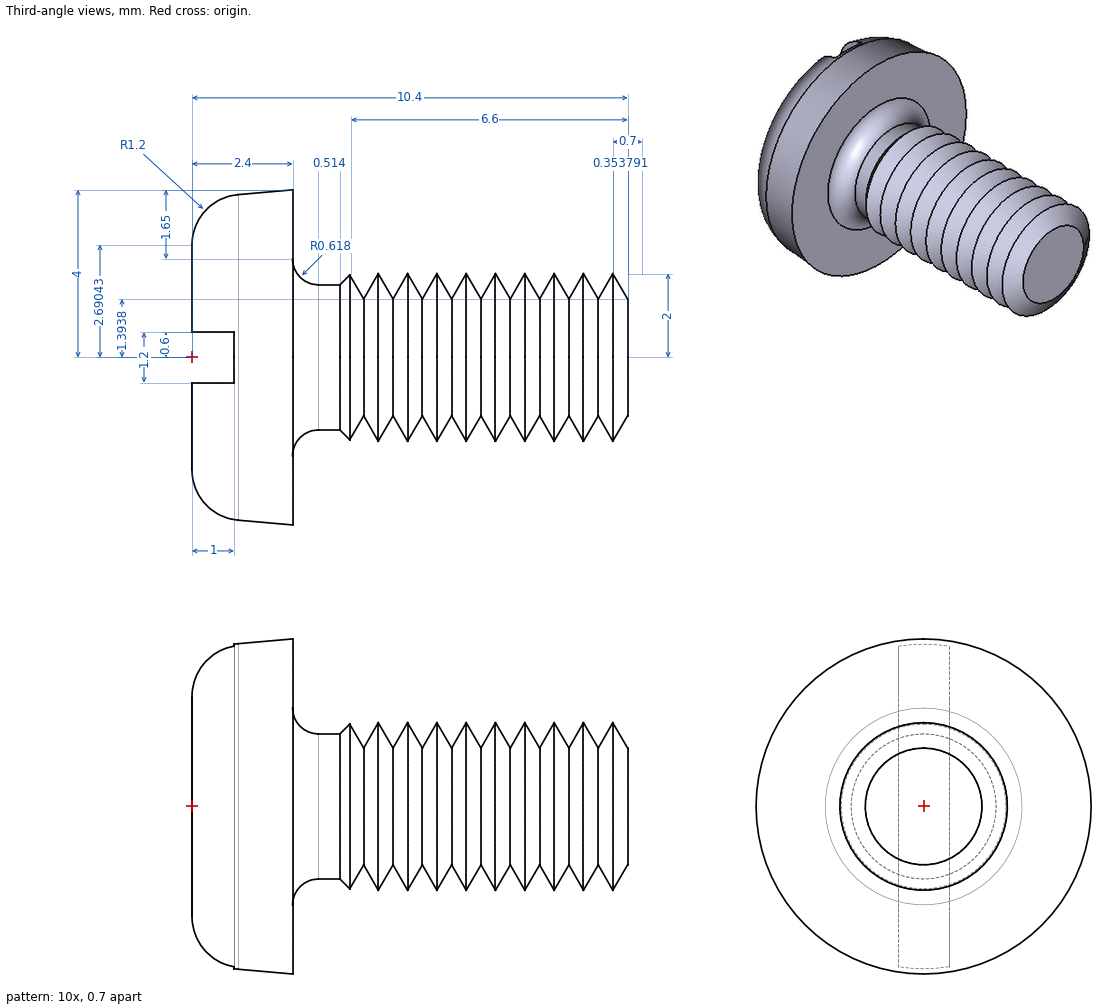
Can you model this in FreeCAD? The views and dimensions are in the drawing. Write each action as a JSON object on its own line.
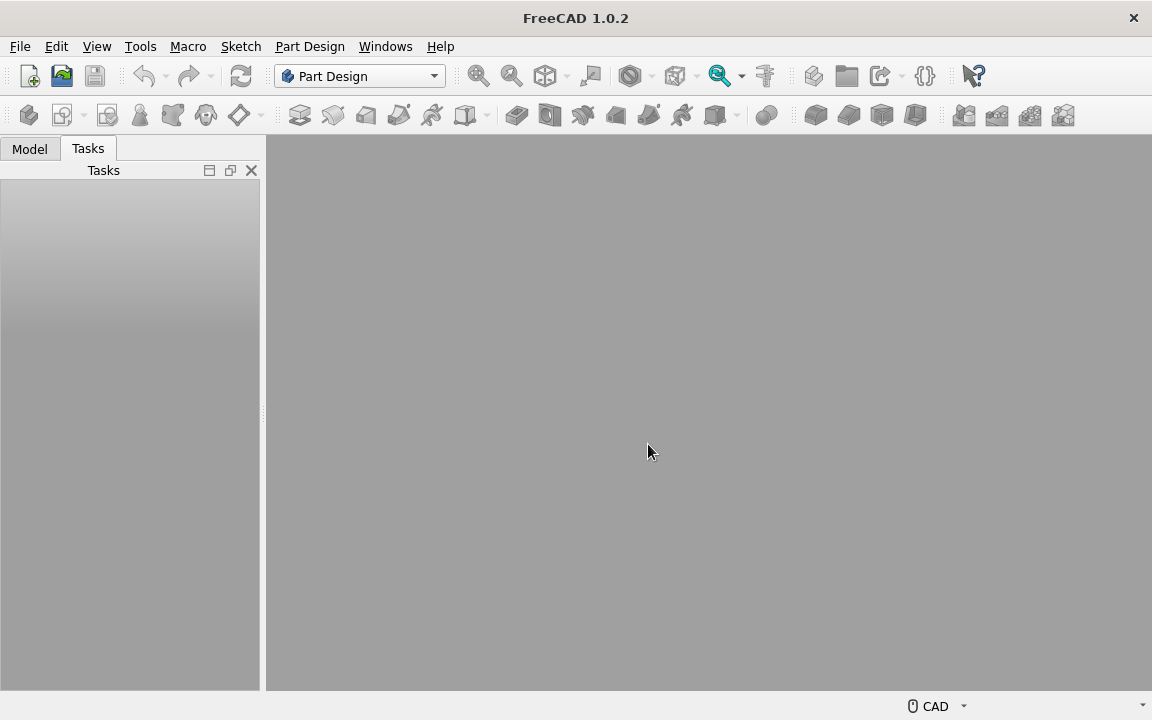
{"action": "left_click", "coordinate": [29, 76]}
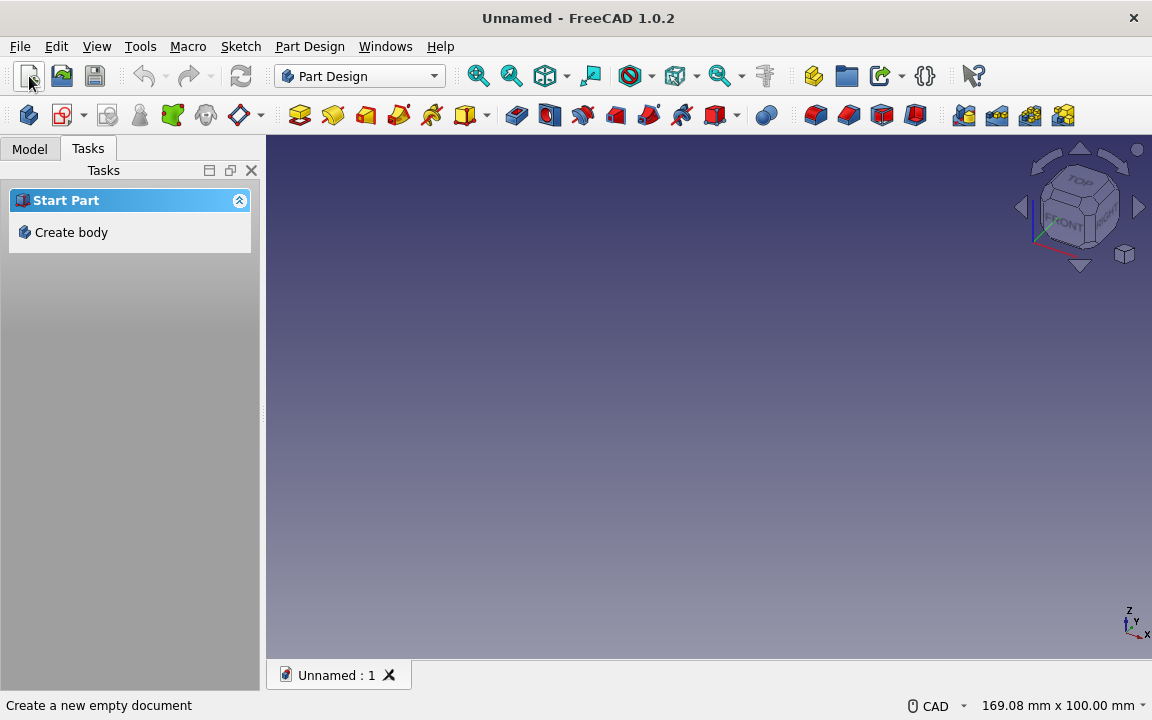
{"action": "left_click", "coordinate": [62, 116]}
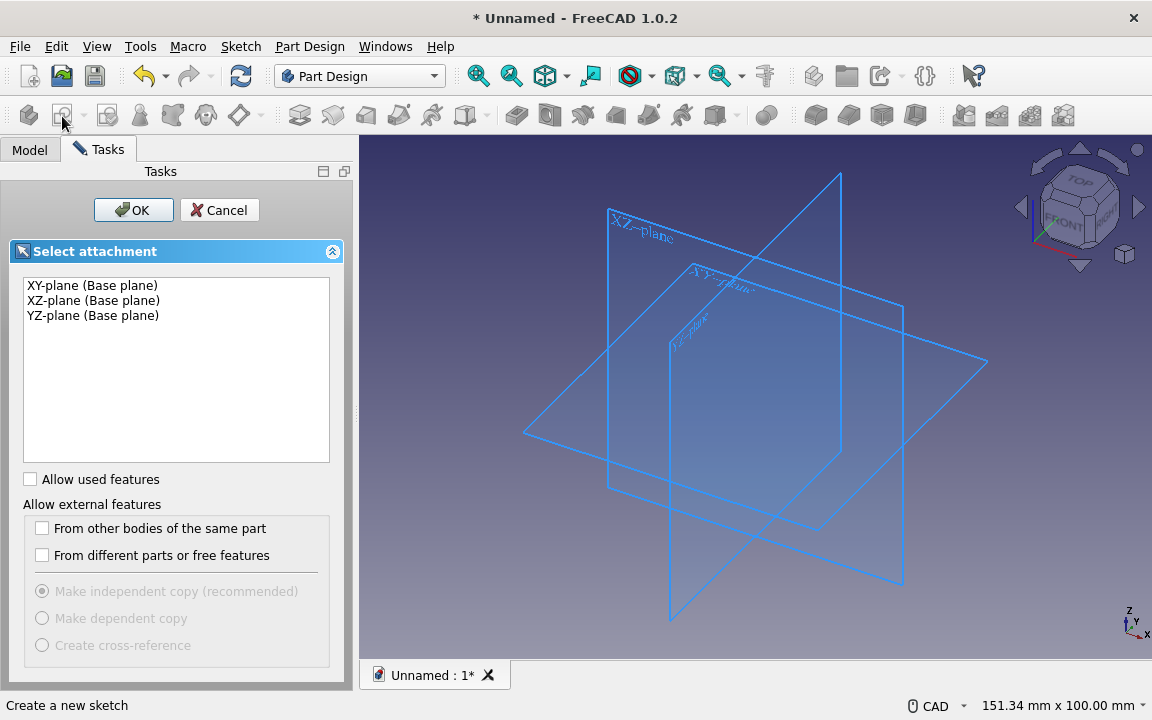
{"action": "left_click", "coordinate": [84, 286]}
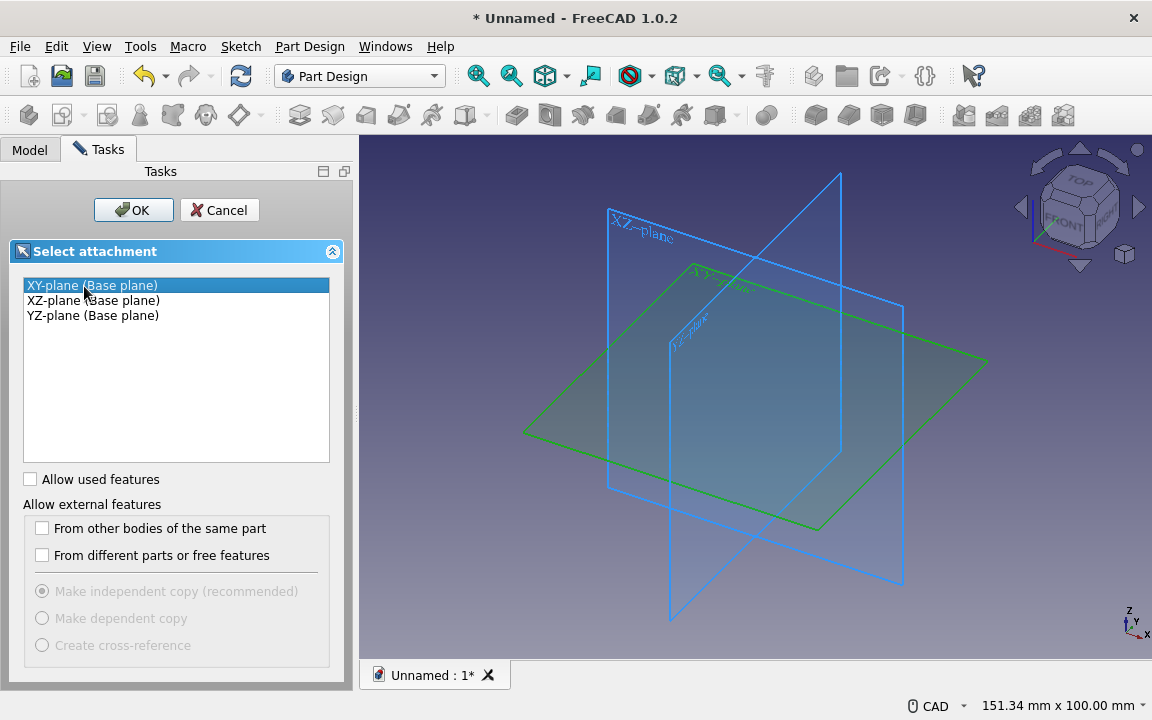
{"action": "left_click", "coordinate": [134, 210]}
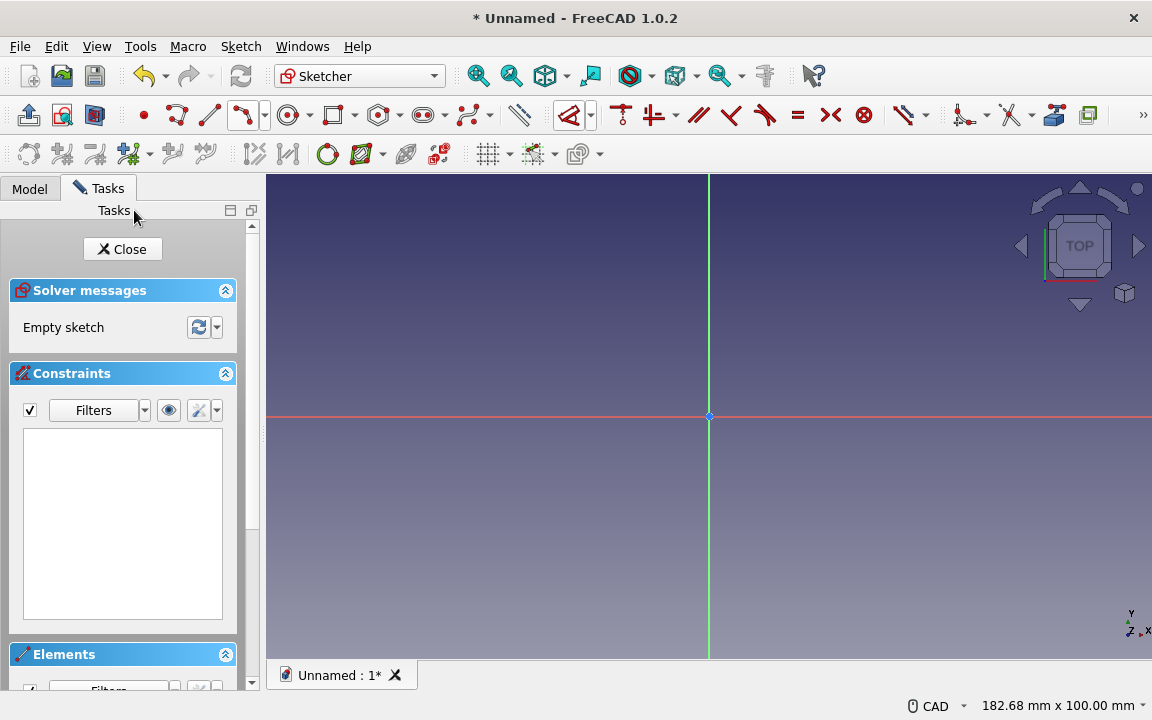
{"action": "scroll", "coordinate": [746, 406], "scroll_direction": "up", "scroll_amount": 11}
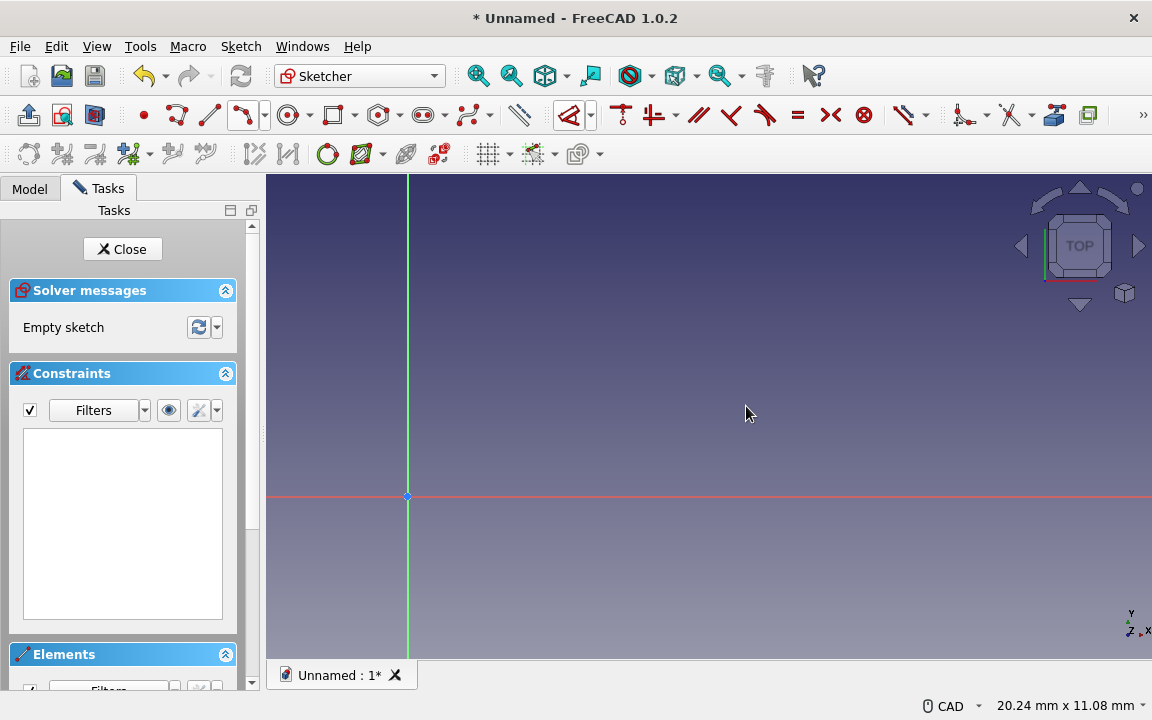
{"action": "left_click", "coordinate": [177, 116]}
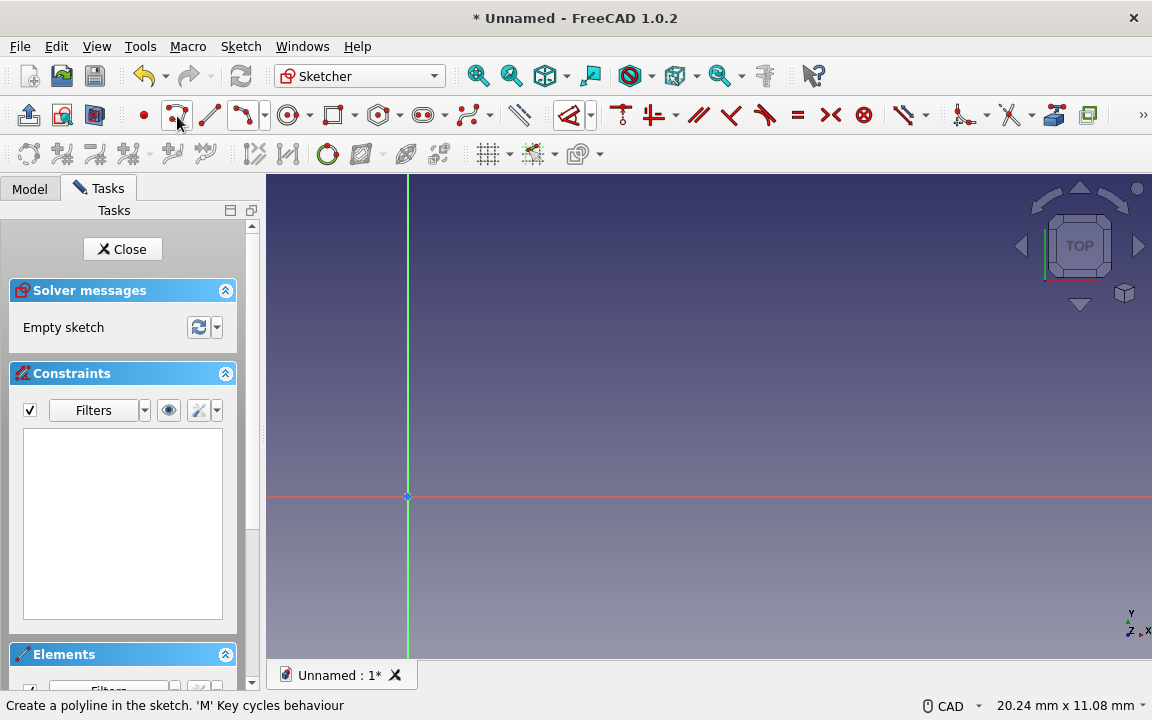
{"action": "left_click", "coordinate": [513, 394]}
{"action": "left_click", "coordinate": [513, 322]}
{"action": "left_click", "coordinate": [456, 327]}
{"action": "right_click", "coordinate": [456, 327]}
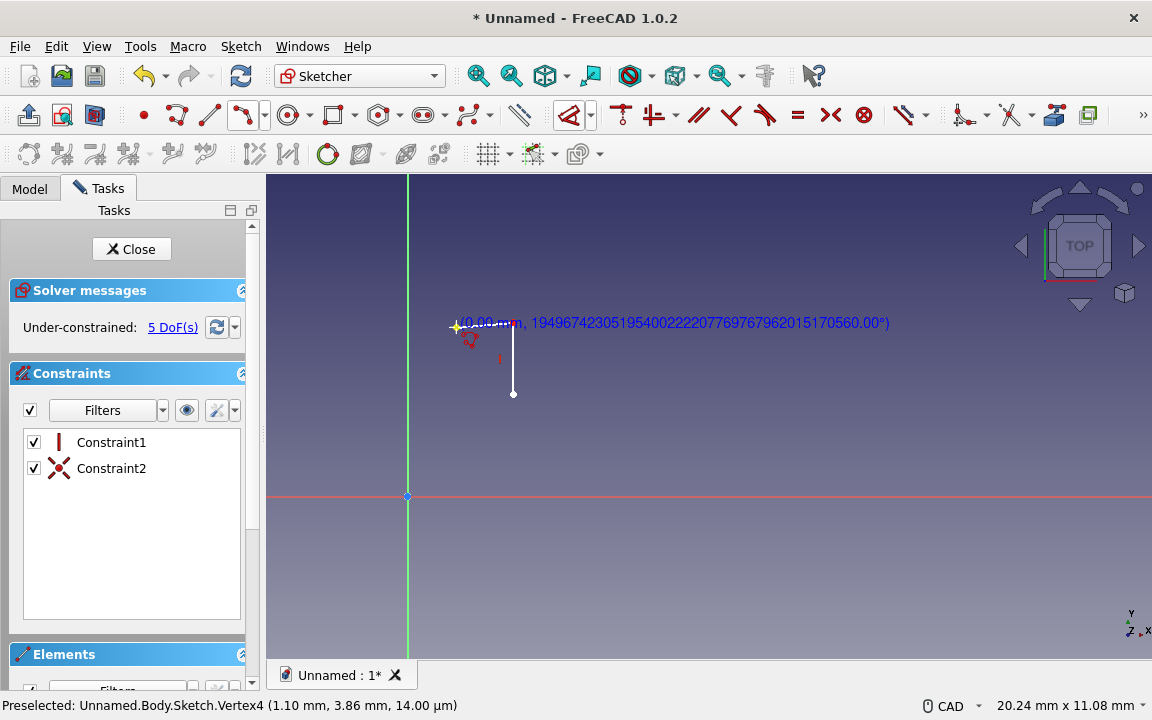
{"action": "left_click", "coordinate": [408, 379]}
{"action": "left_click", "coordinate": [408, 497]}
{"action": "left_click", "coordinate": [863, 488]}
{"action": "left_click", "coordinate": [863, 409]}
{"action": "left_click", "coordinate": [574, 409]}
{"action": "left_click", "coordinate": [562, 421]}
{"action": "left_click", "coordinate": [540, 421]}
{"action": "right_click", "coordinate": [540, 421]}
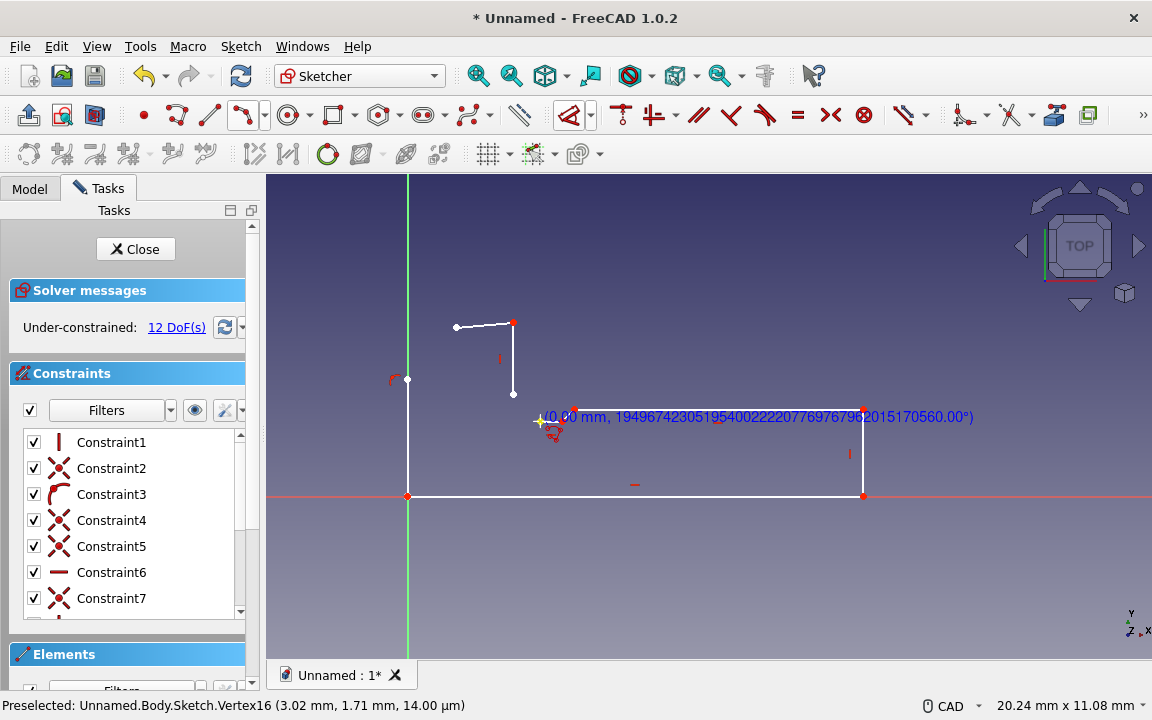
{"action": "left_click", "coordinate": [242, 116]}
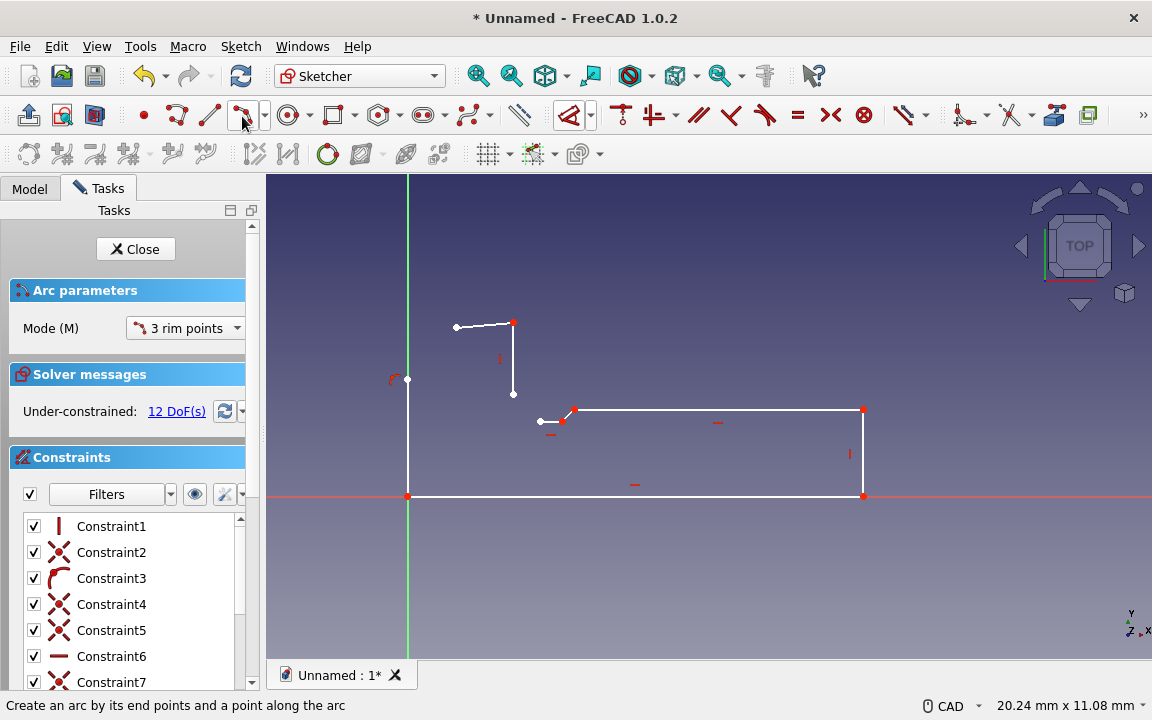
{"action": "left_click", "coordinate": [456, 328]}
{"action": "left_click", "coordinate": [408, 380]}
{"action": "left_click", "coordinate": [422, 344]}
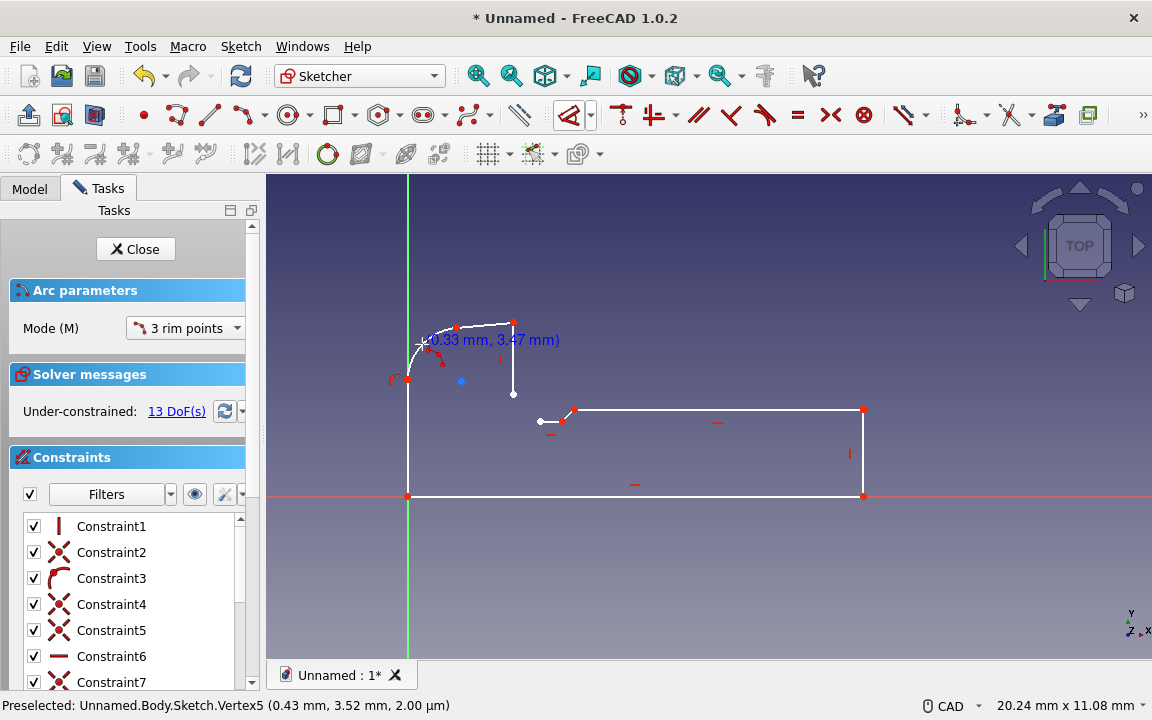
{"action": "scroll", "coordinate": [540, 421], "scroll_direction": "up", "scroll_amount": 2}